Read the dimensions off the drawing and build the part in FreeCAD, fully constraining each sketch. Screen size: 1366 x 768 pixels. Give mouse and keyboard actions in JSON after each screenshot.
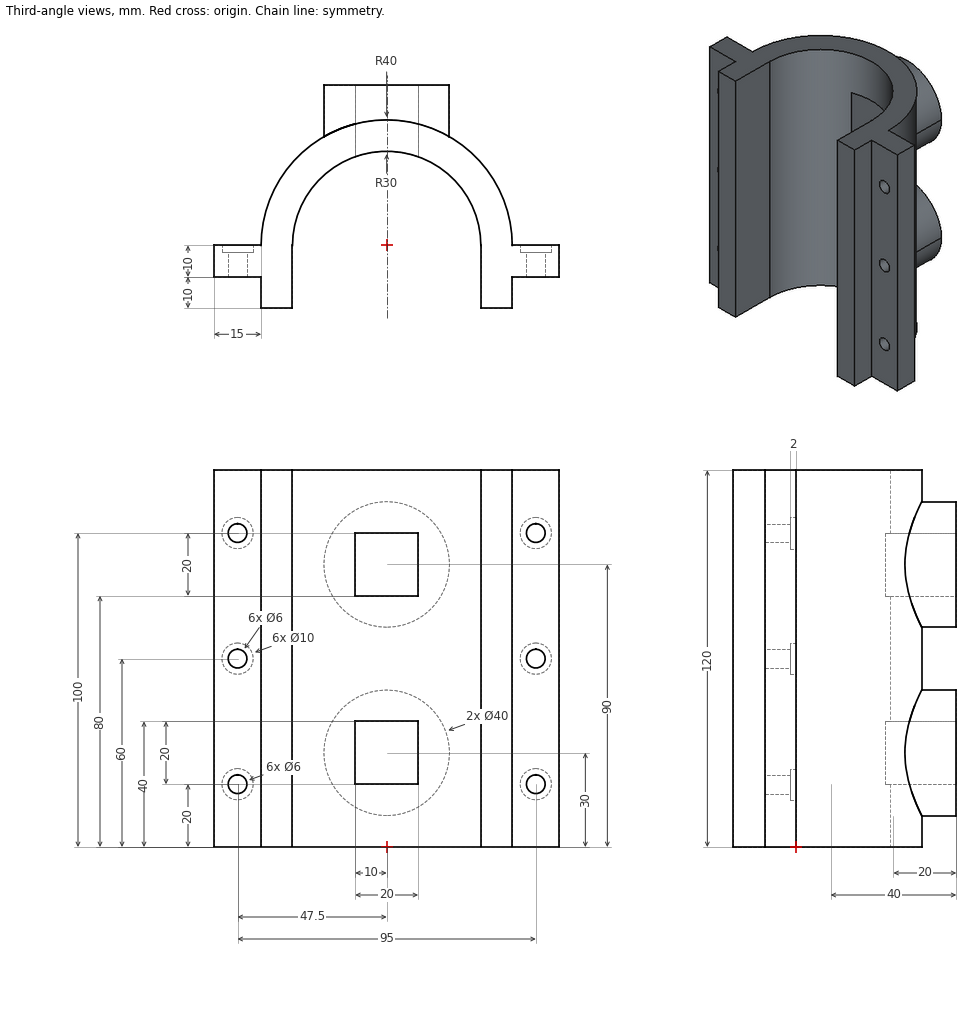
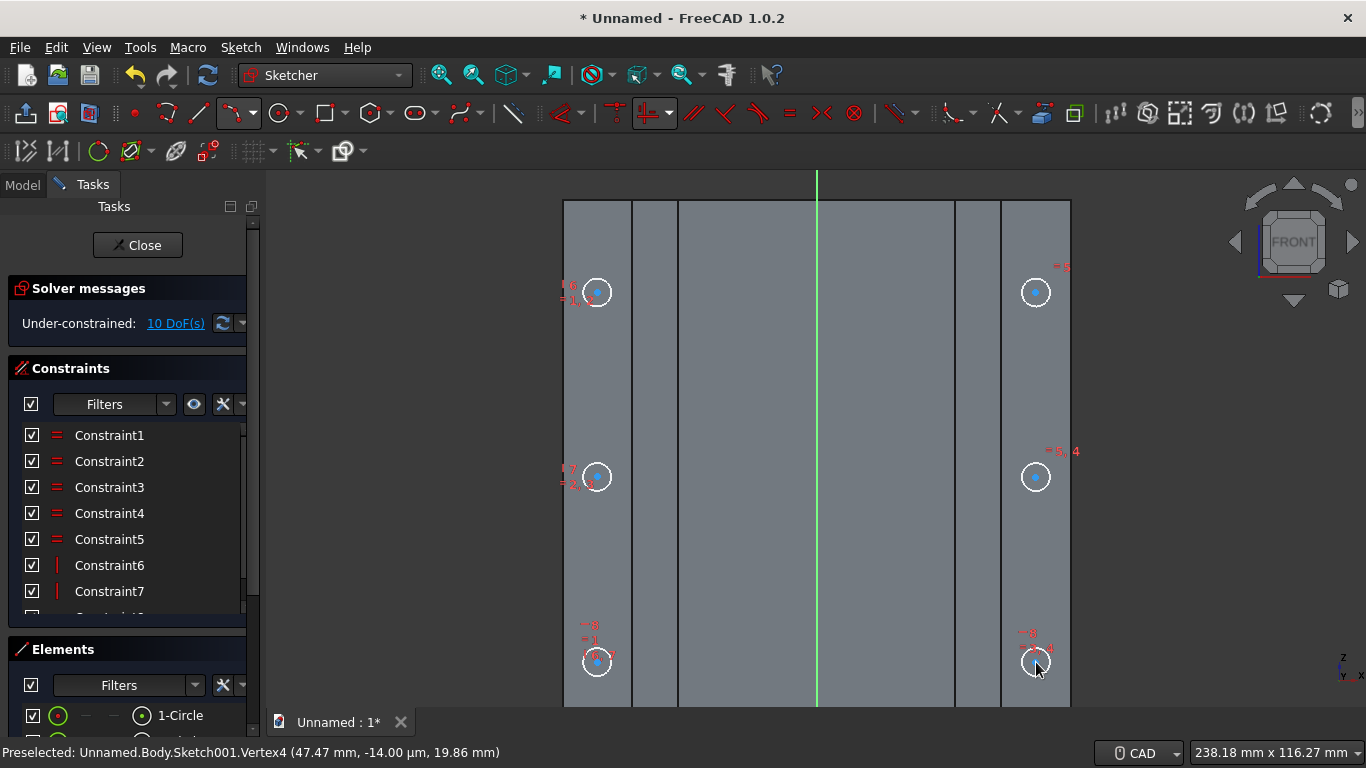
{"action": "left_click", "coordinate": [1036, 662]}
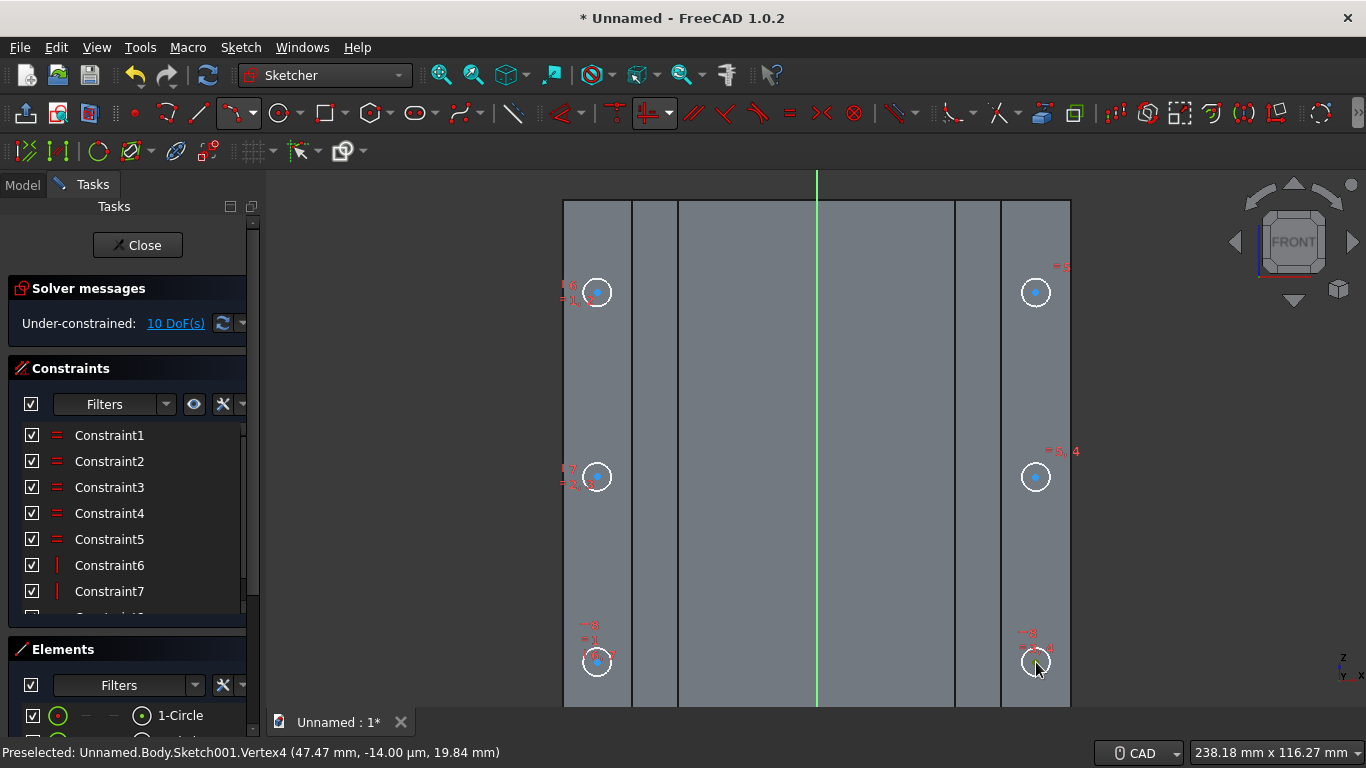
{"action": "left_click", "coordinate": [1036, 477]}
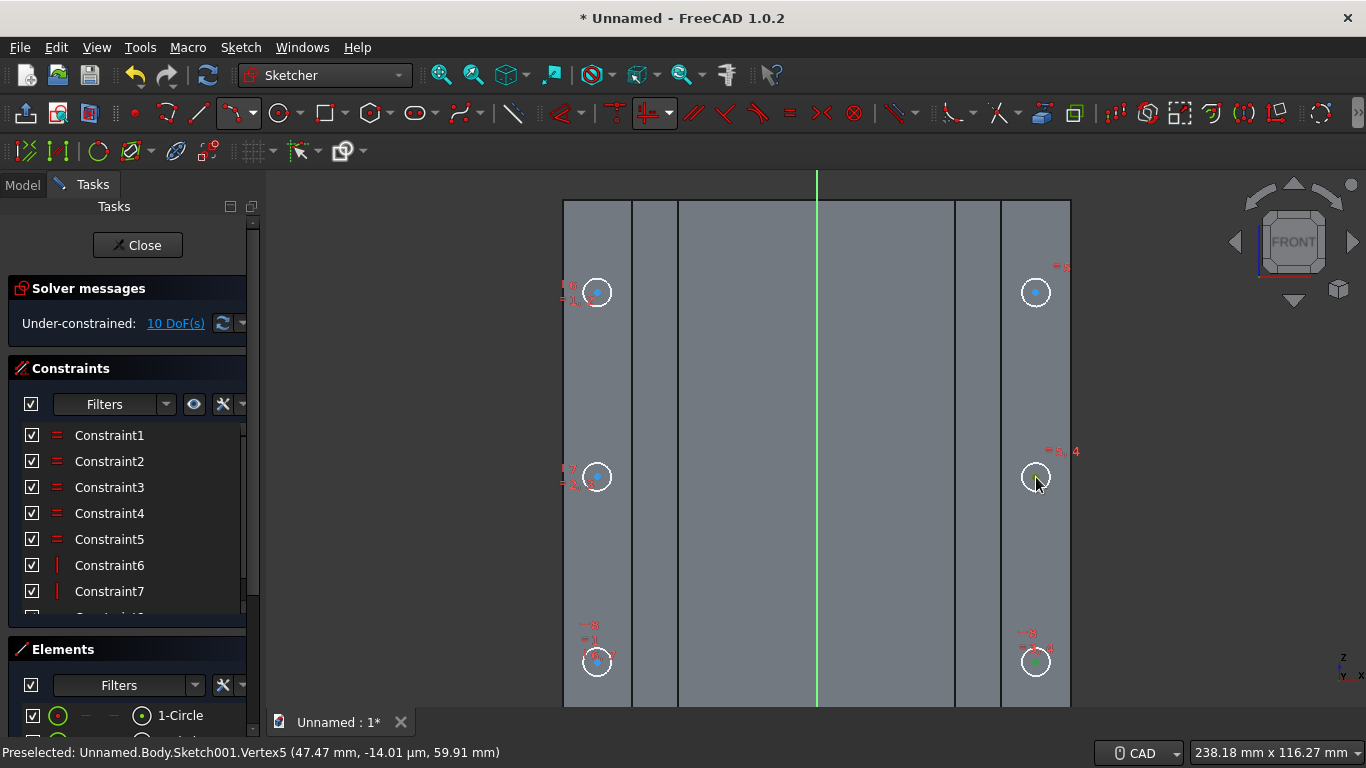
{"action": "key", "text": "v"}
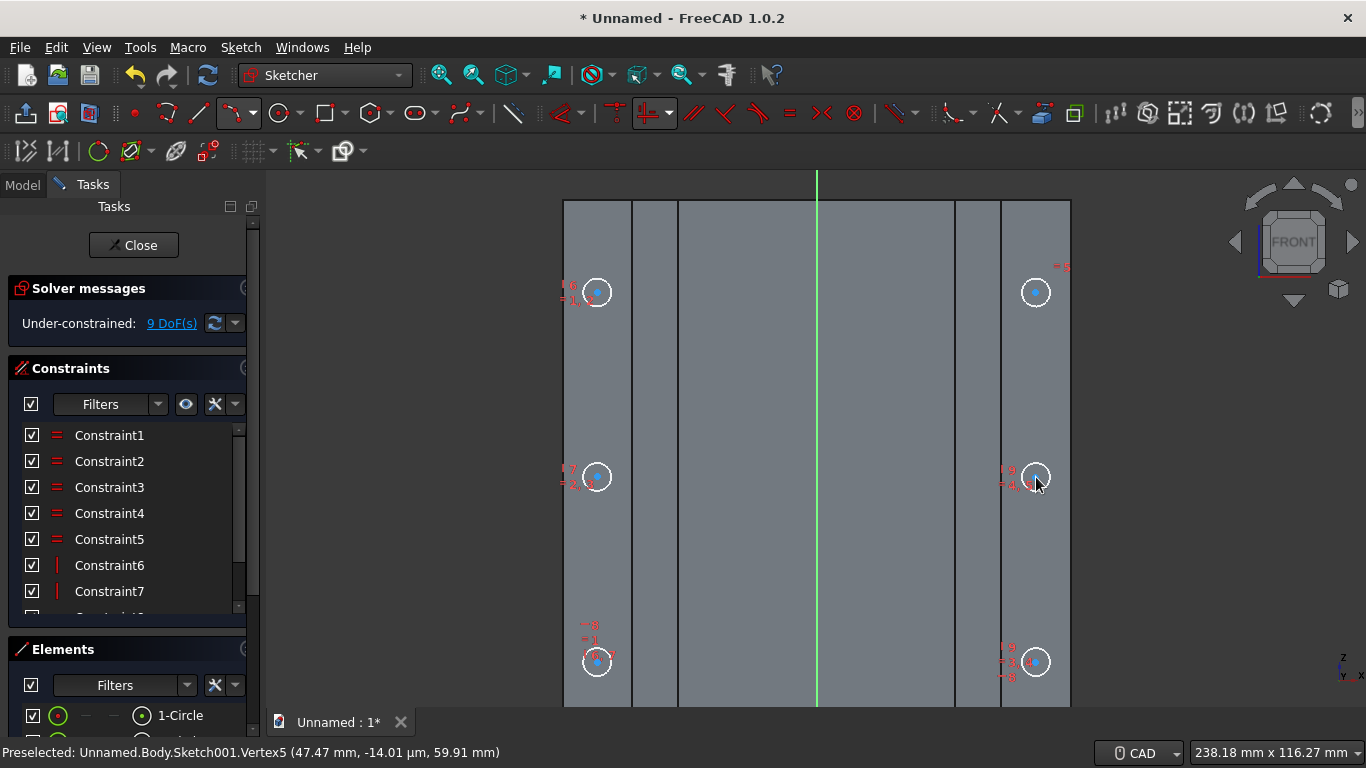
{"action": "left_click", "coordinate": [597, 477]}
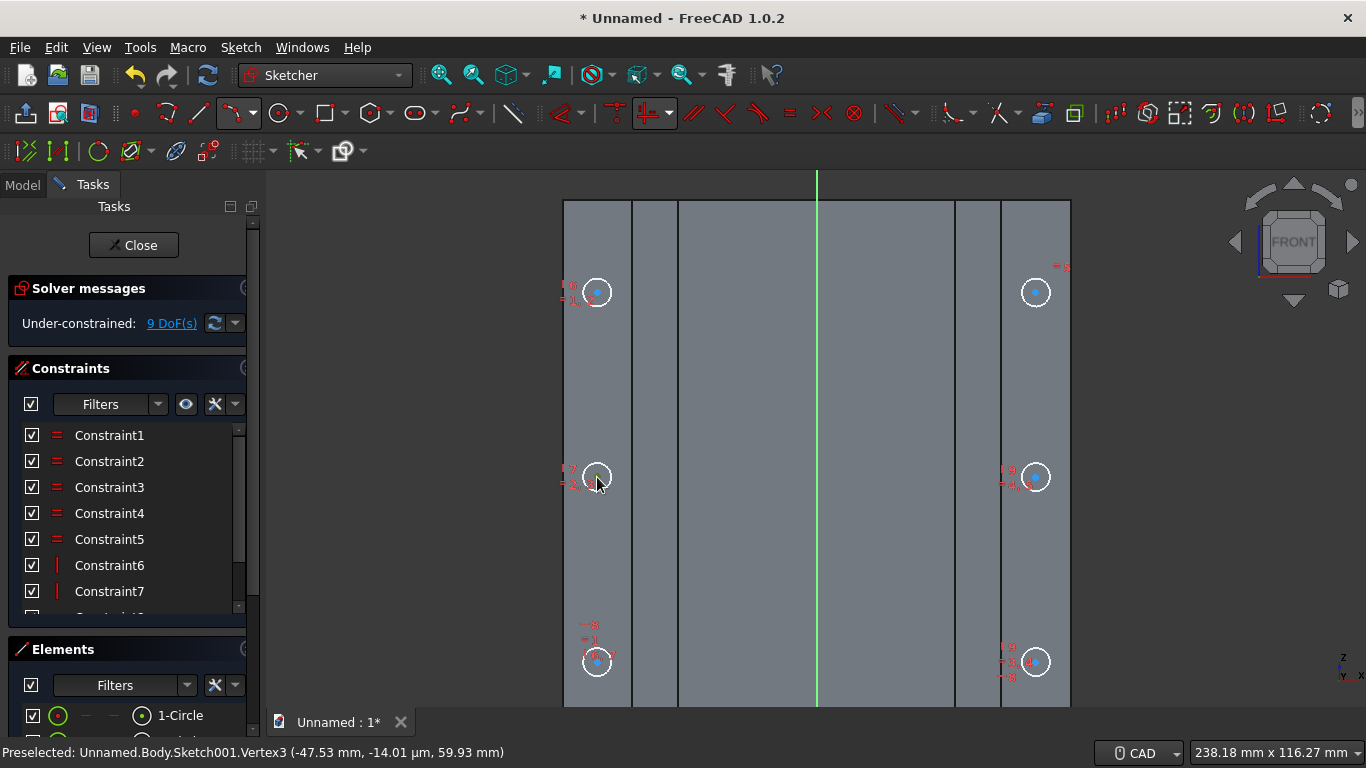
{"action": "left_click", "coordinate": [1036, 477]}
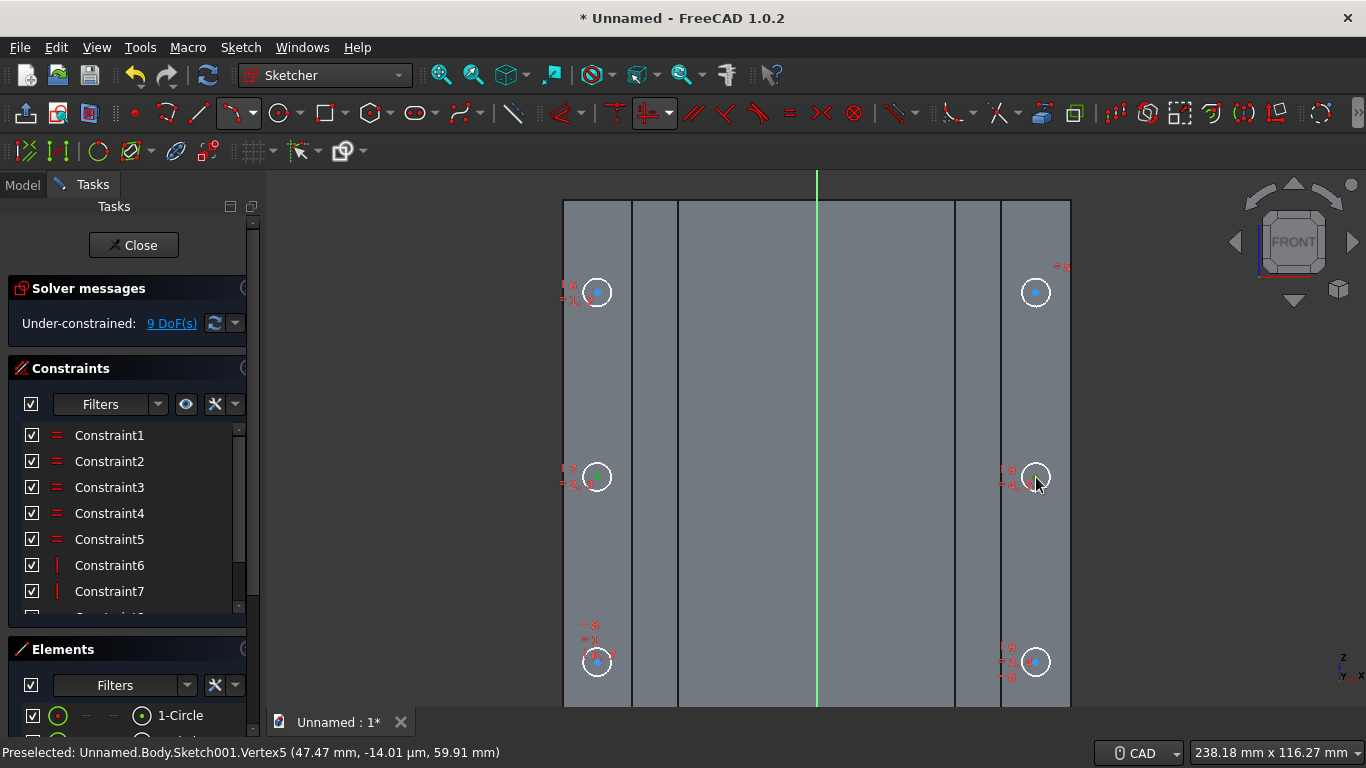
{"action": "left_click", "coordinate": [672, 114]}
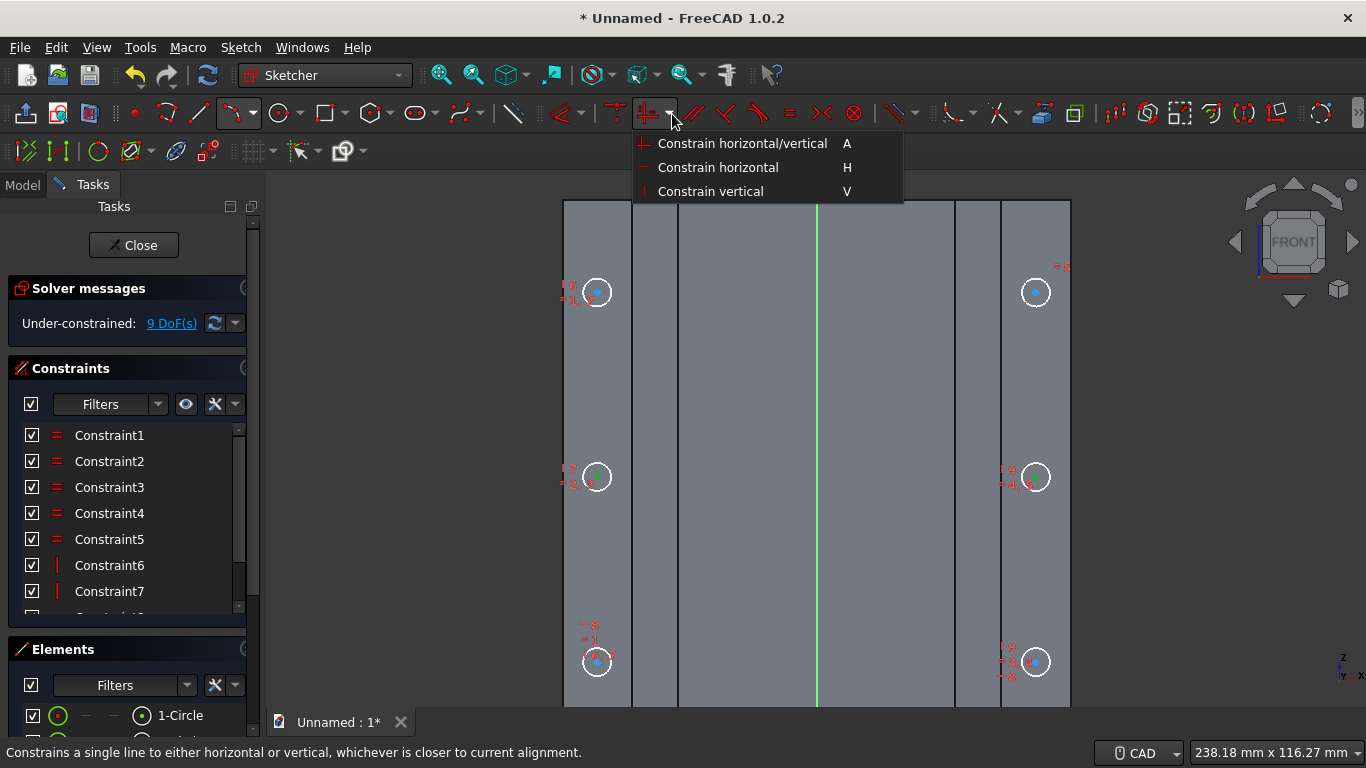
{"action": "left_click", "coordinate": [768, 167]}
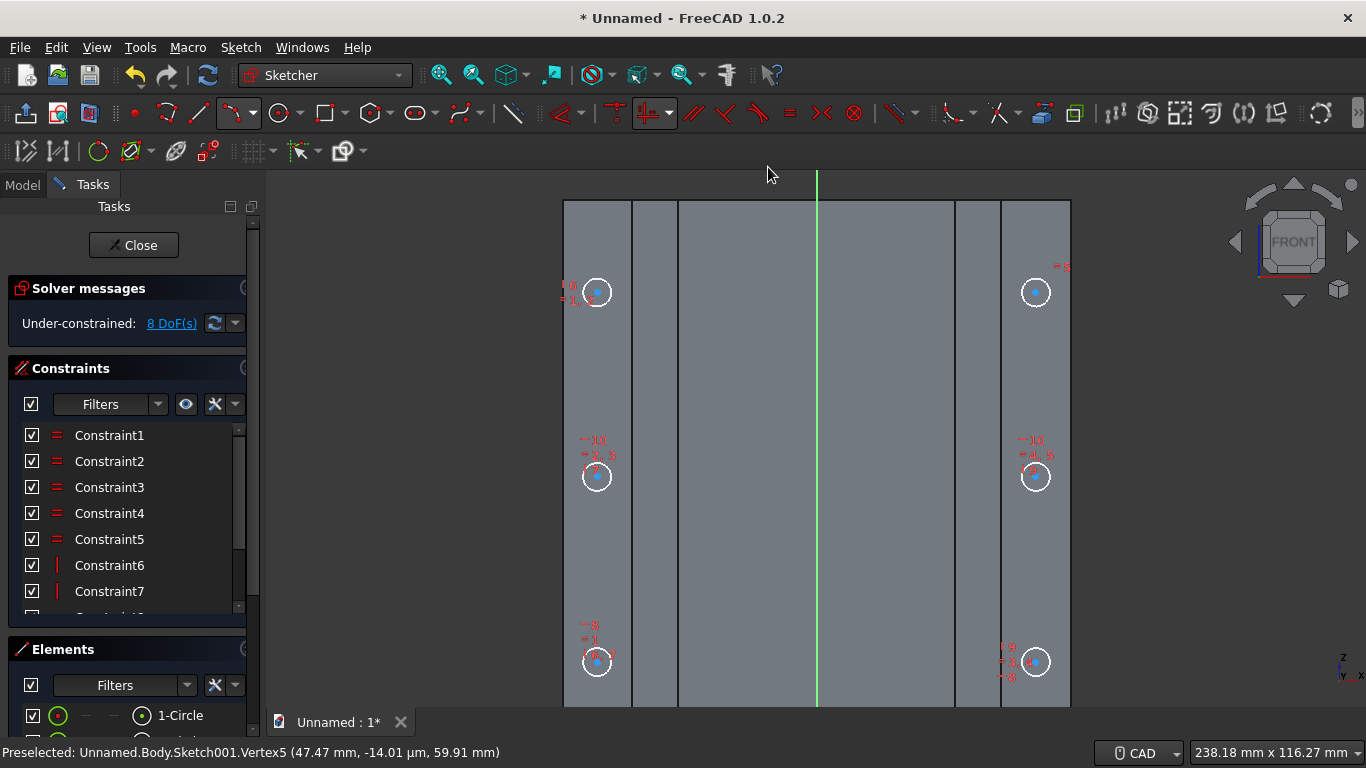
{"action": "left_click", "coordinate": [1036, 477]}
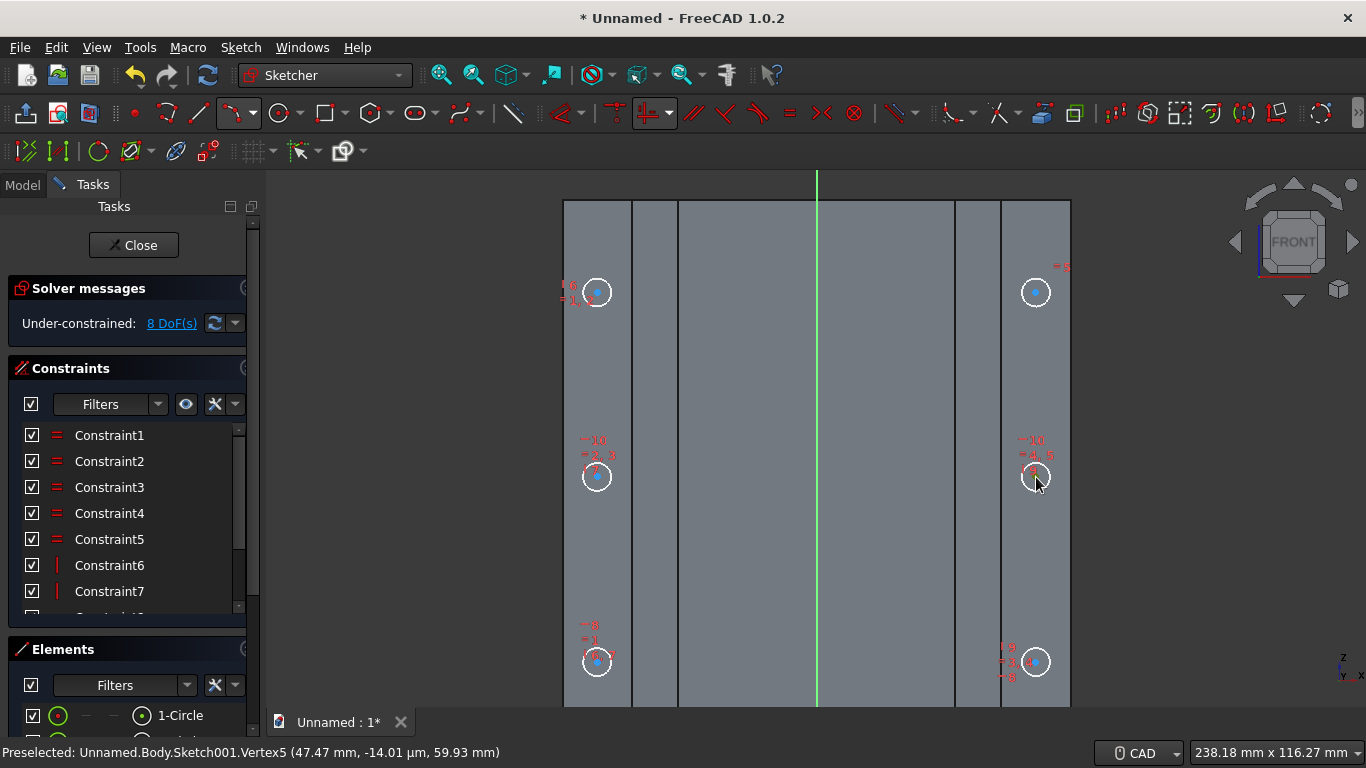
{"action": "left_click", "coordinate": [1036, 293]}